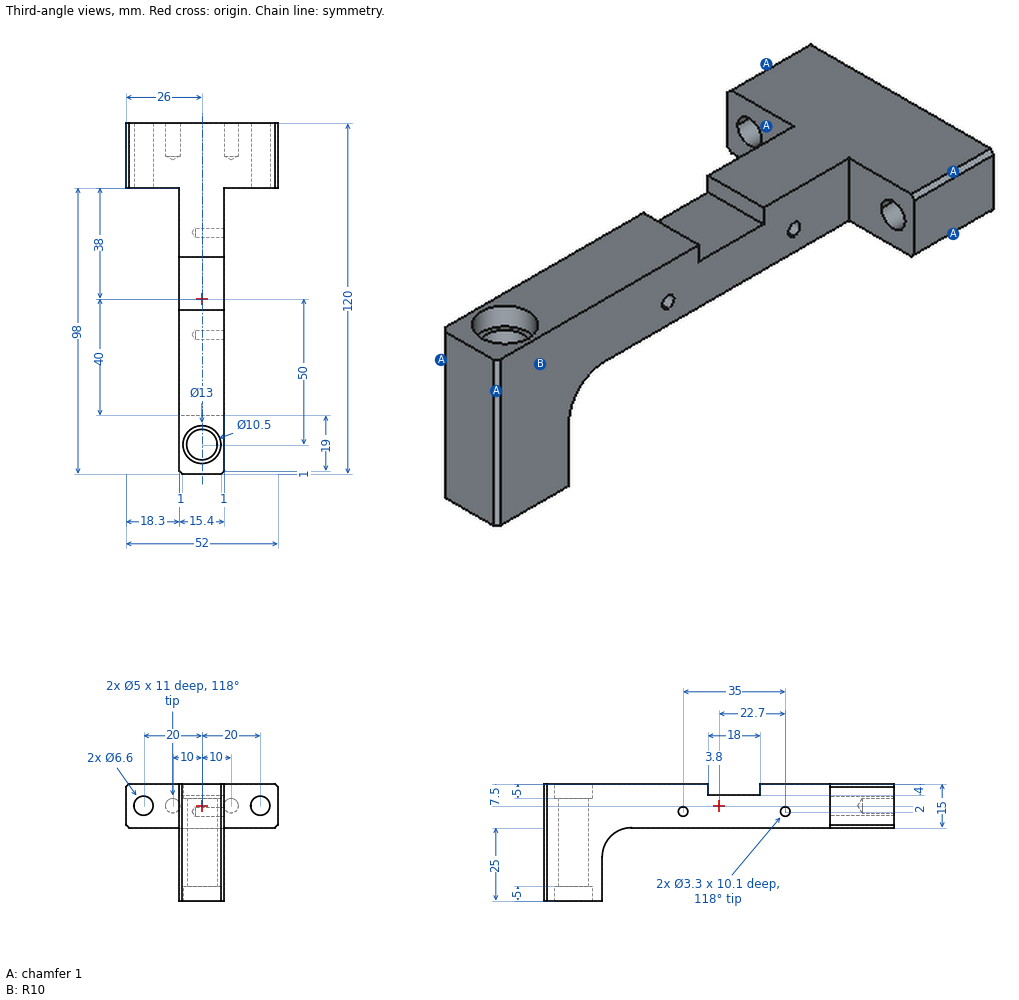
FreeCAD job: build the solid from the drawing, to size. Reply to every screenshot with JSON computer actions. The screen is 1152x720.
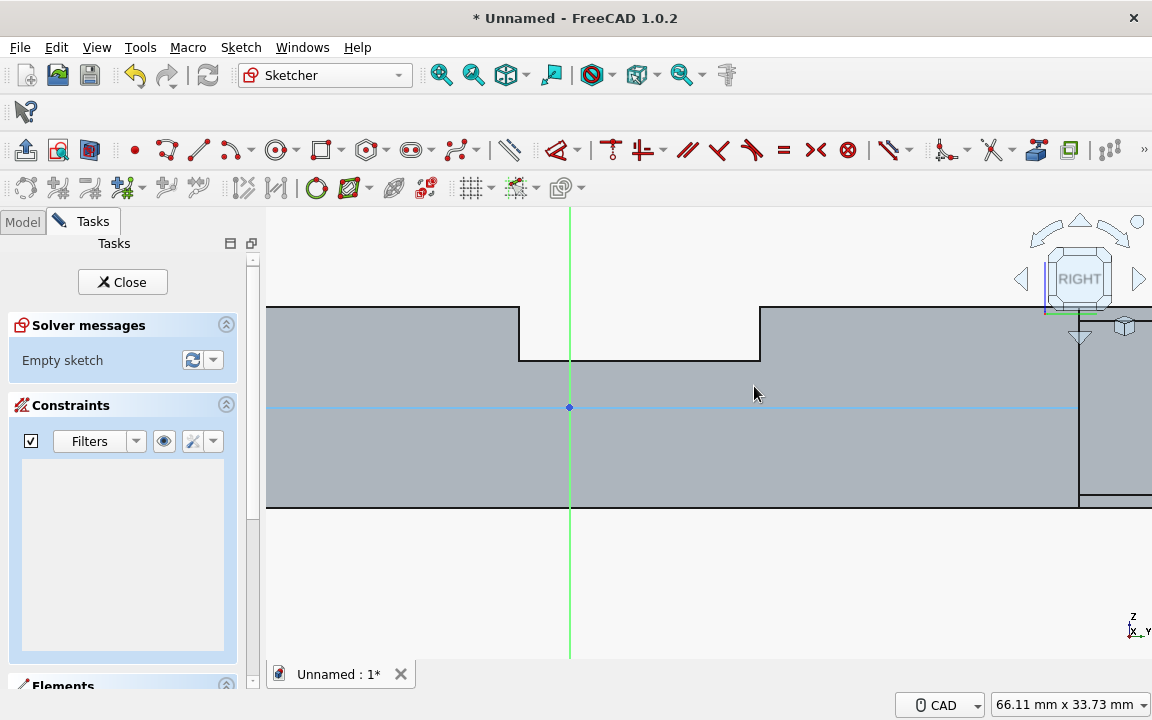
{"action": "left_click", "coordinate": [276, 150]}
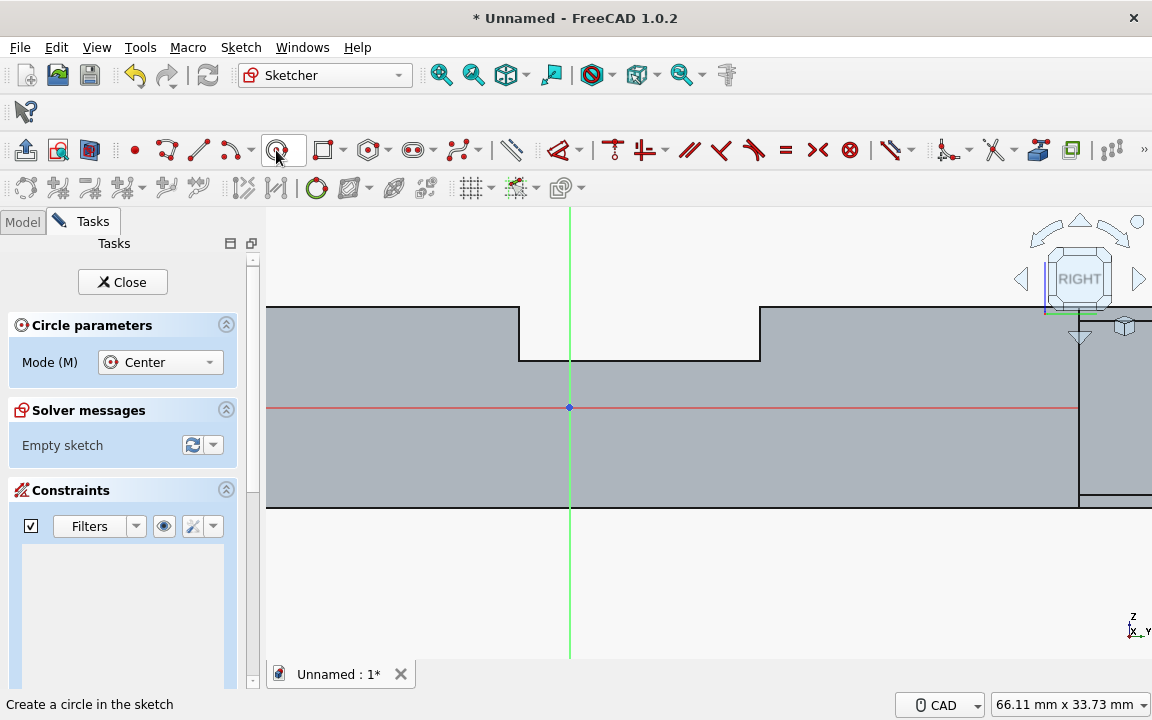
{"action": "left_click", "coordinate": [874, 435]}
{"action": "mouse_move", "coordinate": [890, 450]}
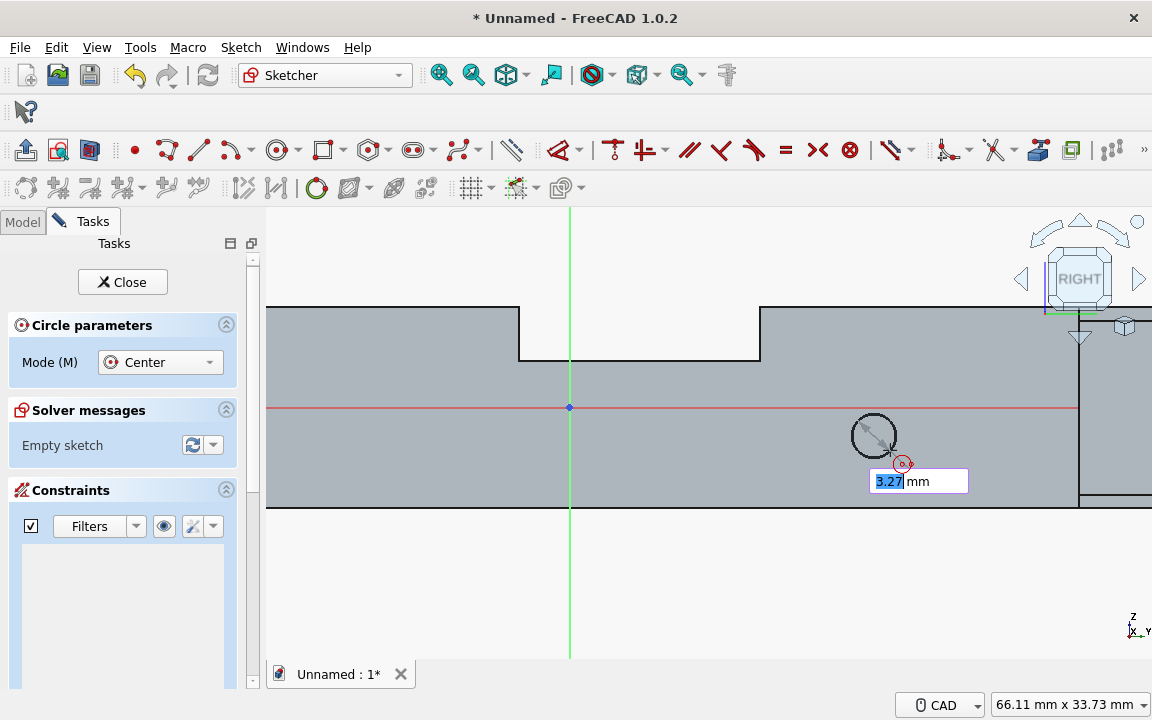
{"action": "type", "text": "3.3"}
{"action": "key", "text": "Return"}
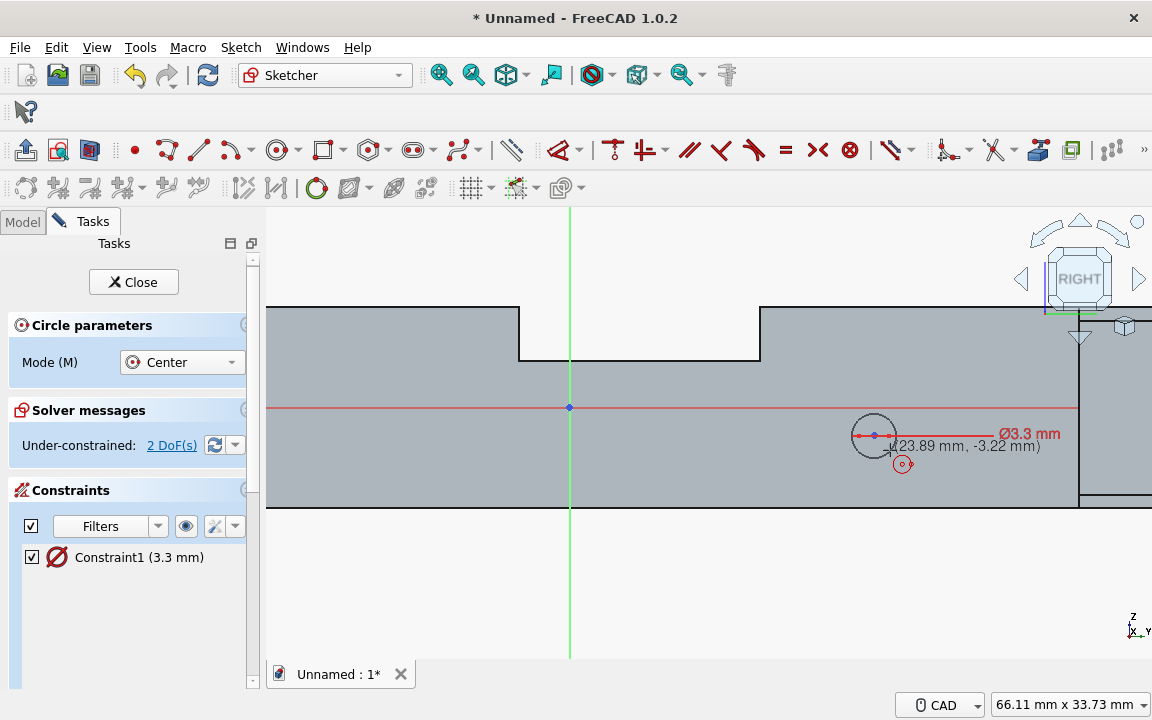
{"action": "left_click", "coordinate": [405, 435]}
{"action": "mouse_move", "coordinate": [421, 450]}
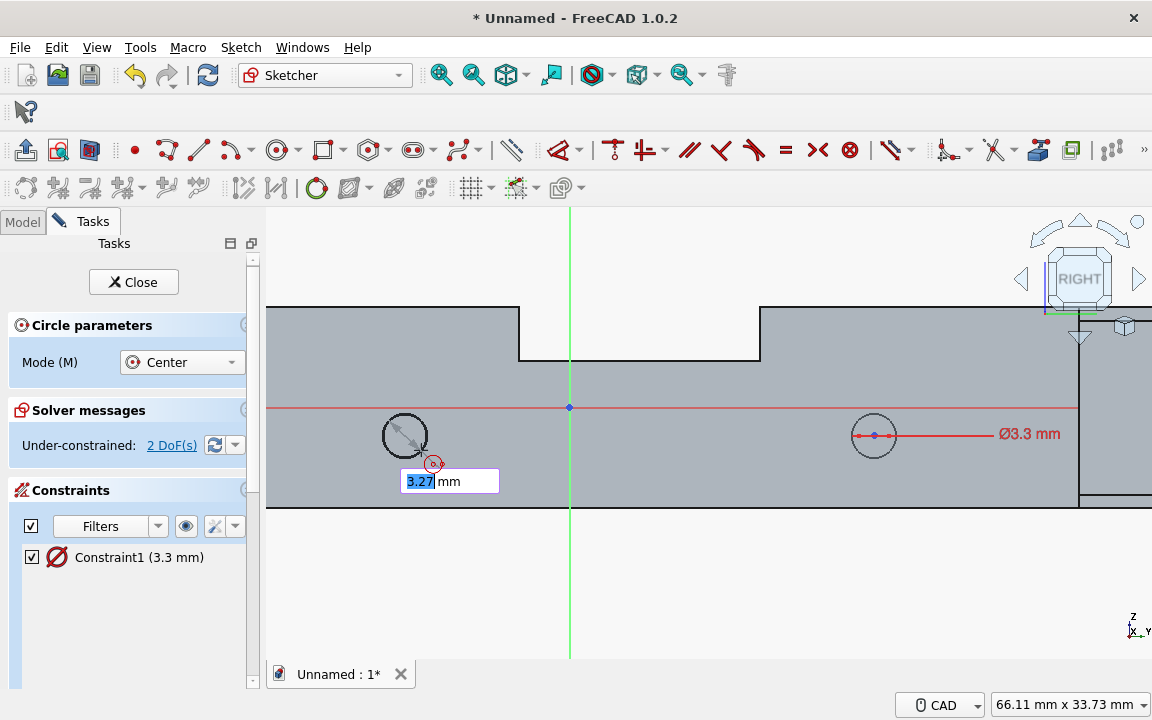
{"action": "type", "text": "3.3"}
{"action": "key", "text": "Return"}
{"action": "key", "text": "Escape"}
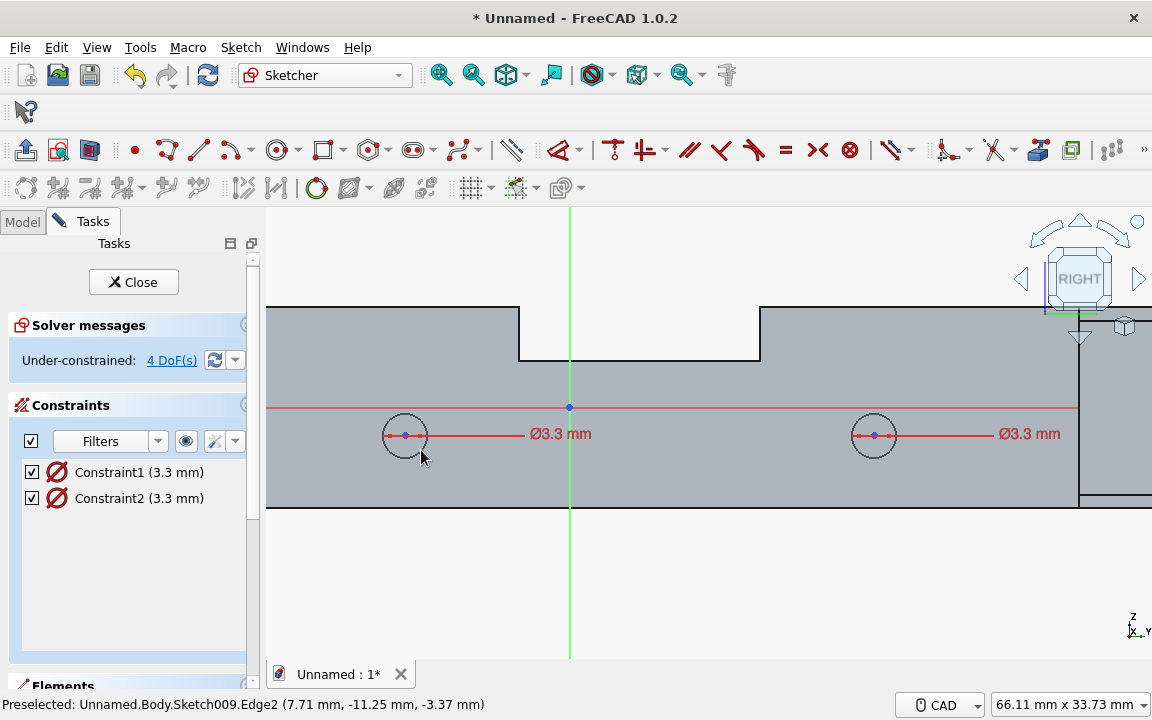
{"action": "left_click", "coordinate": [874, 436]}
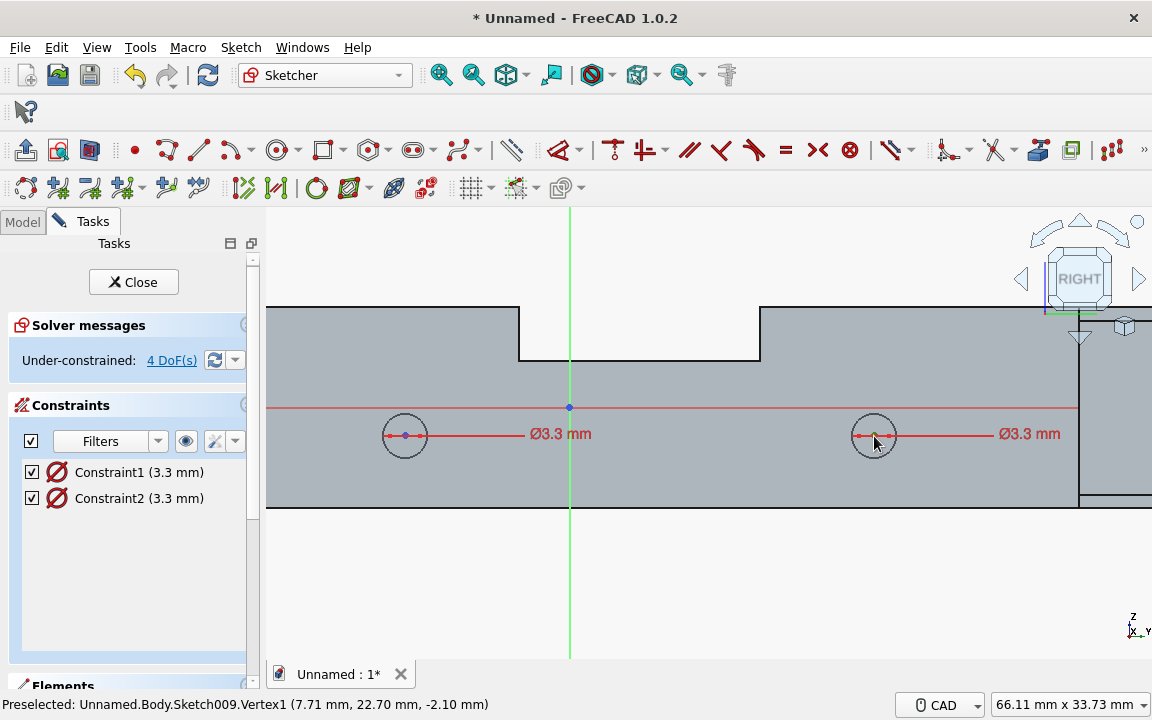
{"action": "left_click", "coordinate": [405, 436]}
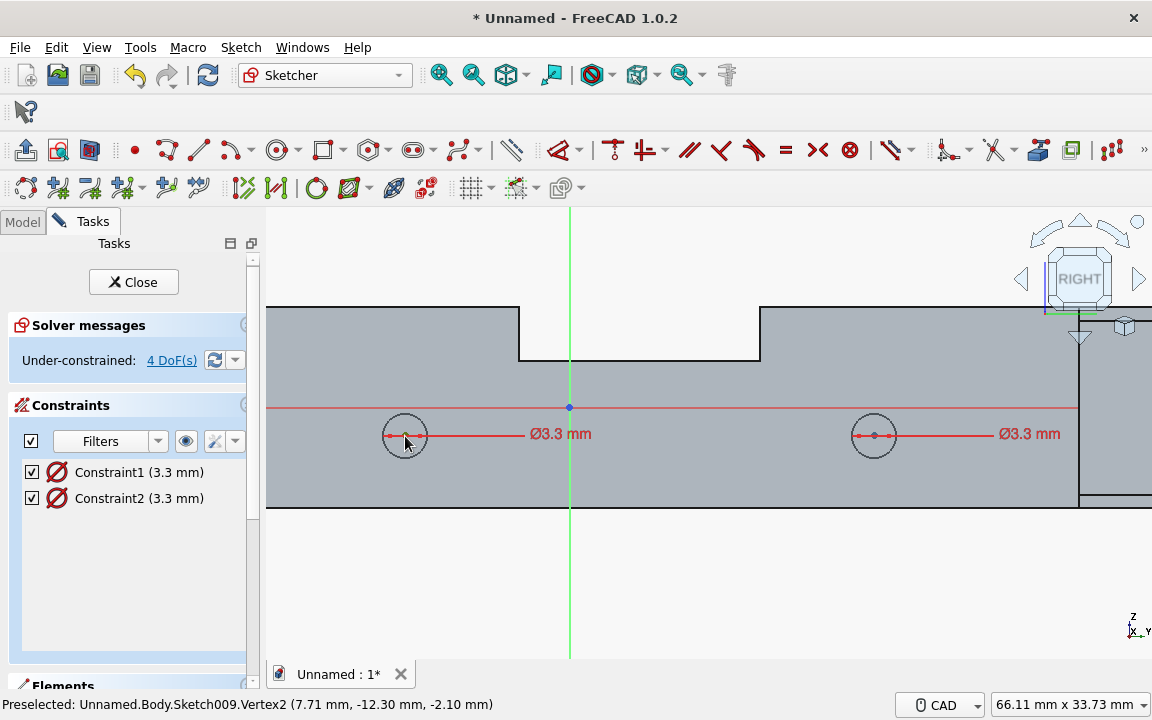
{"action": "key", "text": "h"}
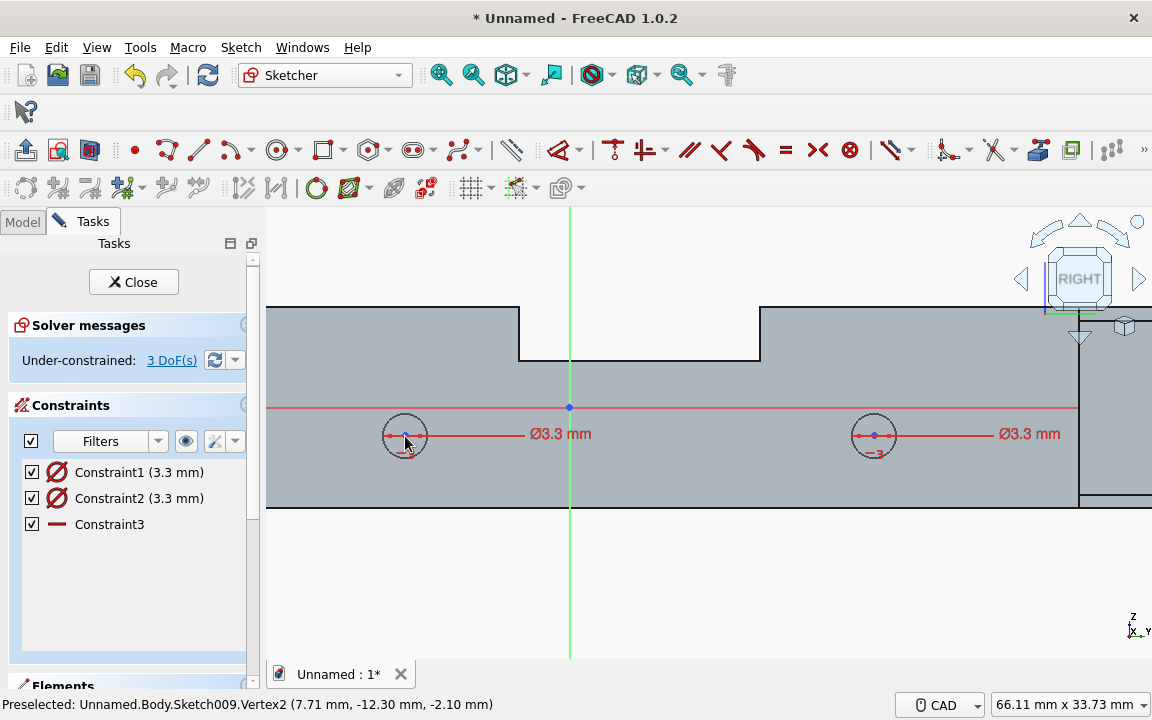
{"action": "left_click", "coordinate": [558, 150]}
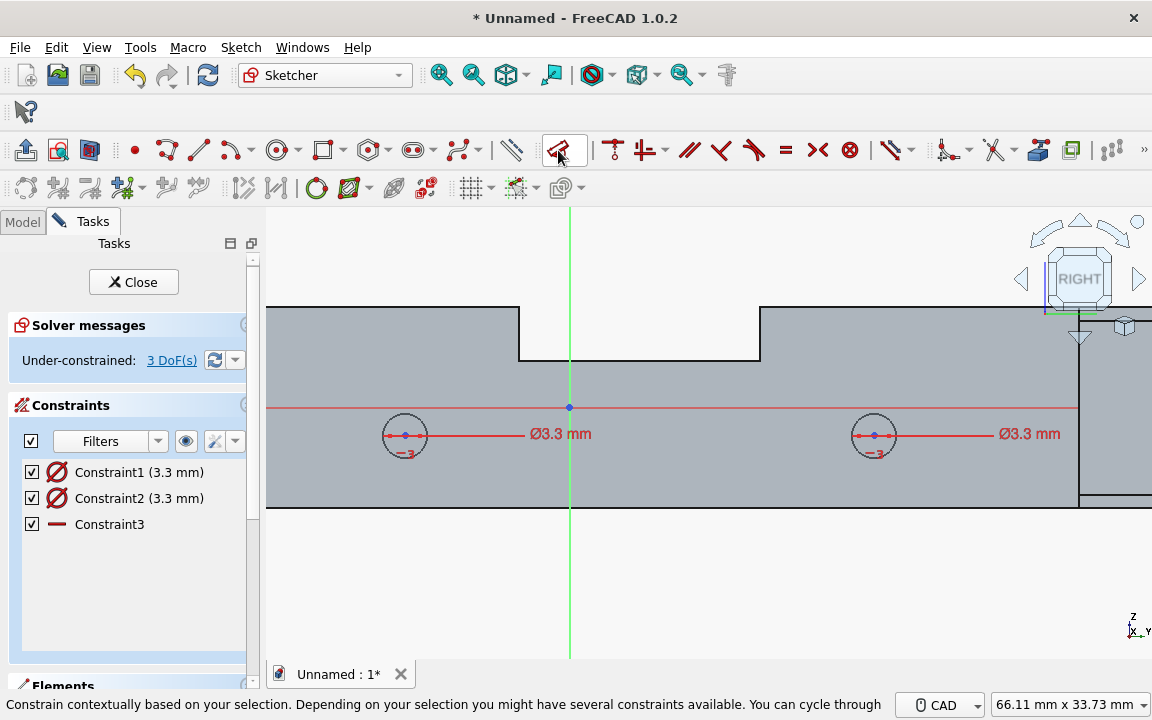
{"action": "scroll", "coordinate": [874, 436], "scroll_direction": "up", "scroll_amount": 2}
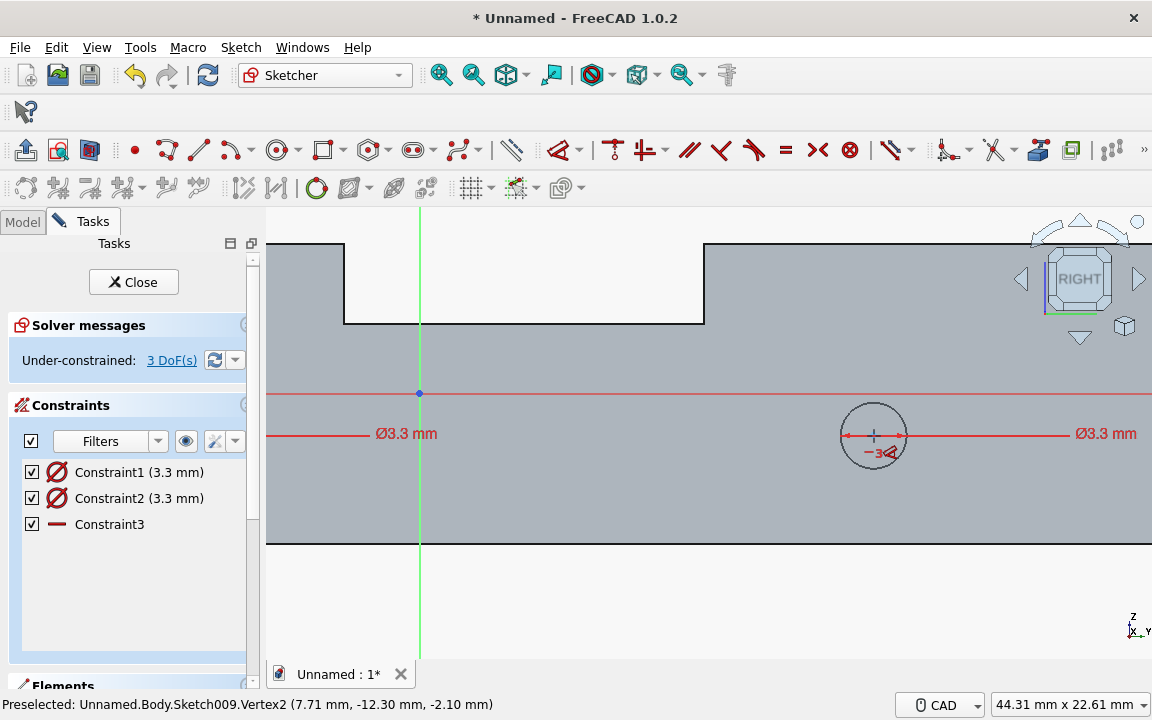
{"action": "left_click", "coordinate": [874, 436]}
{"action": "left_click", "coordinate": [386, 415]}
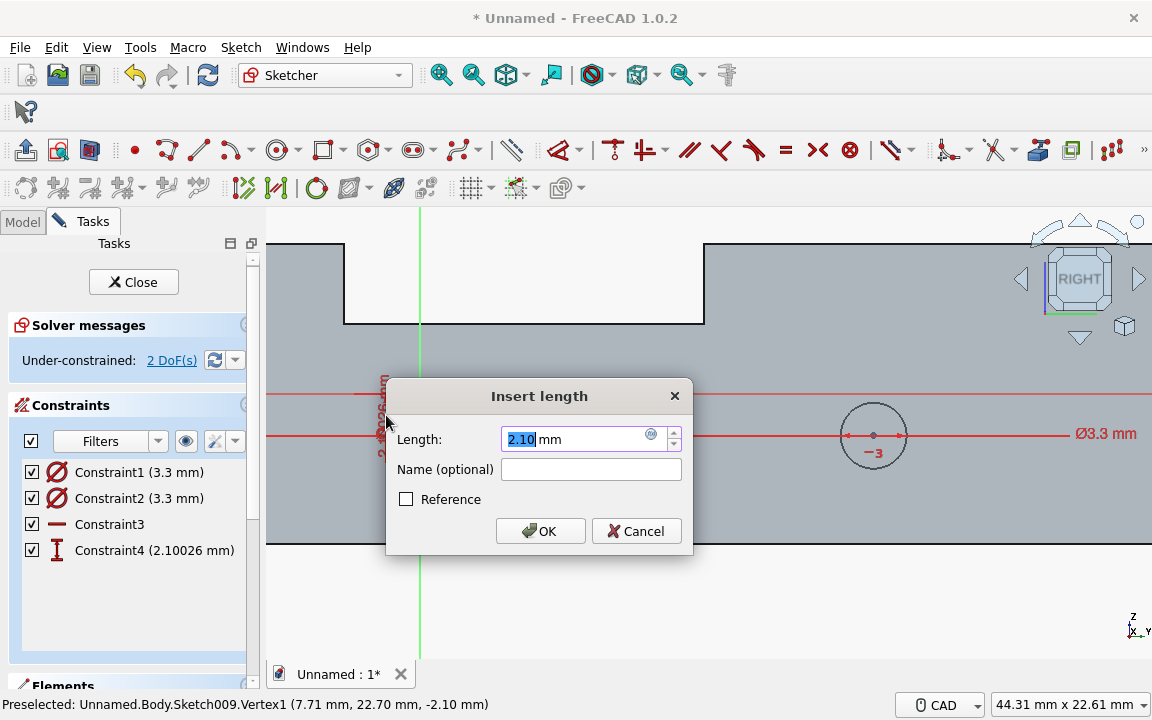
{"action": "type", "text": "2"}
{"action": "key", "text": "Return"}